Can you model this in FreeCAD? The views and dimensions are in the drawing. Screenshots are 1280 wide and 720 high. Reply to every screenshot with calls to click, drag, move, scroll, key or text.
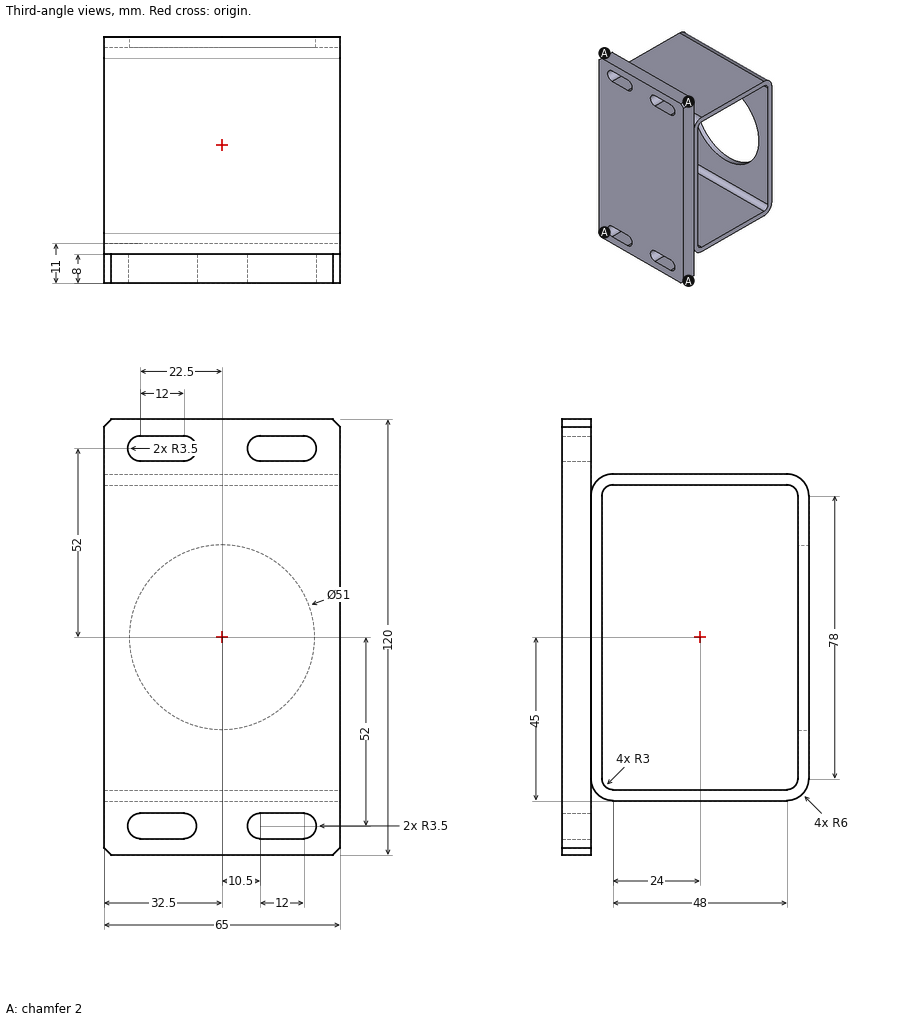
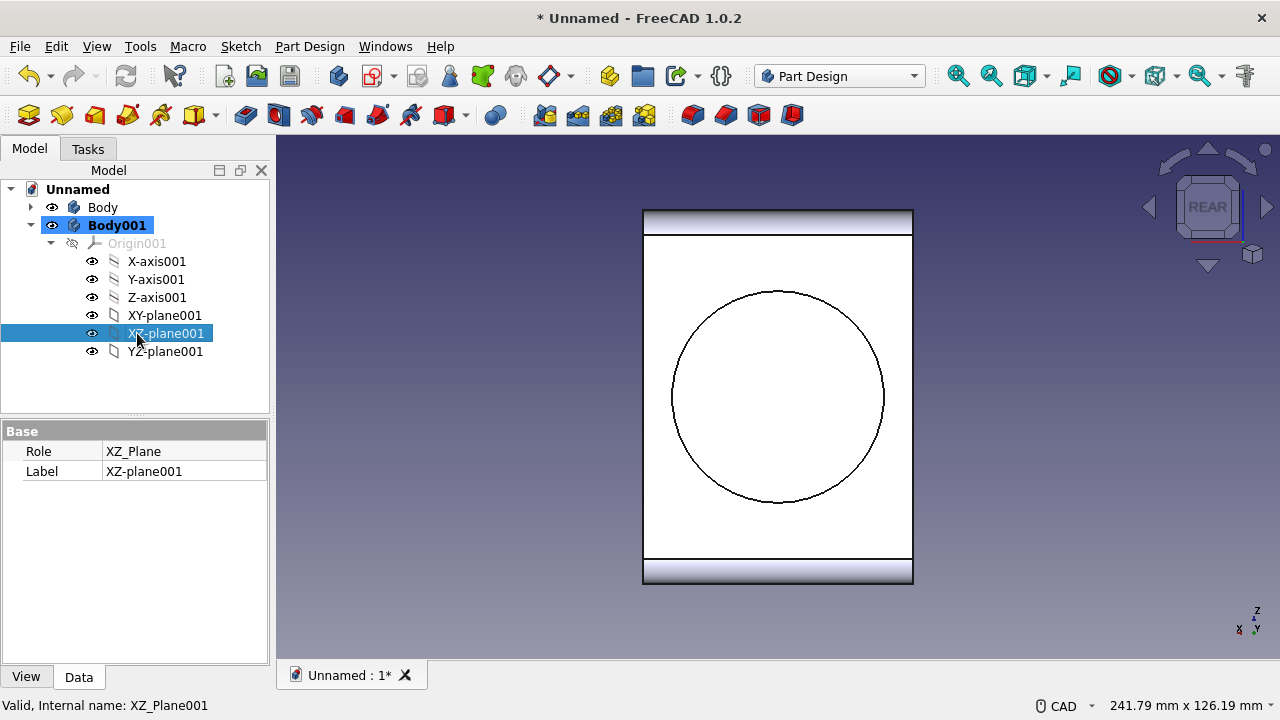
click(548, 76)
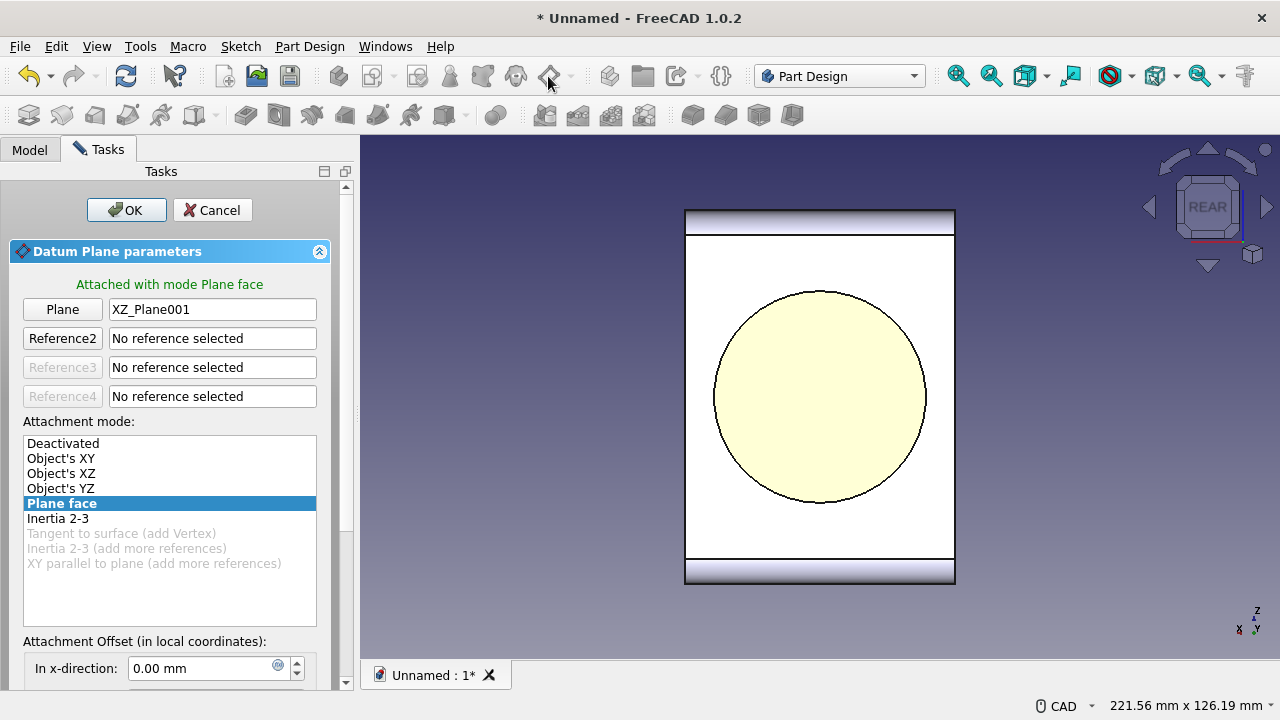
scroll(346, 436, down, 2)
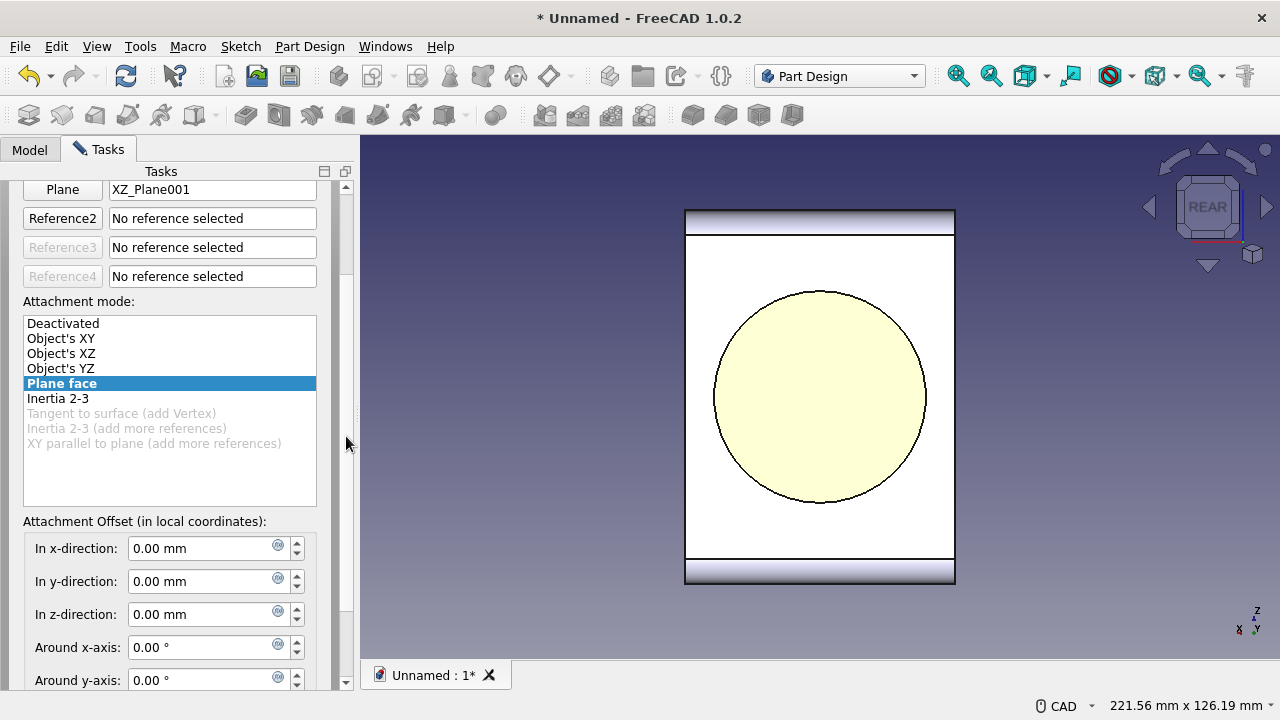
triple_click(210, 614)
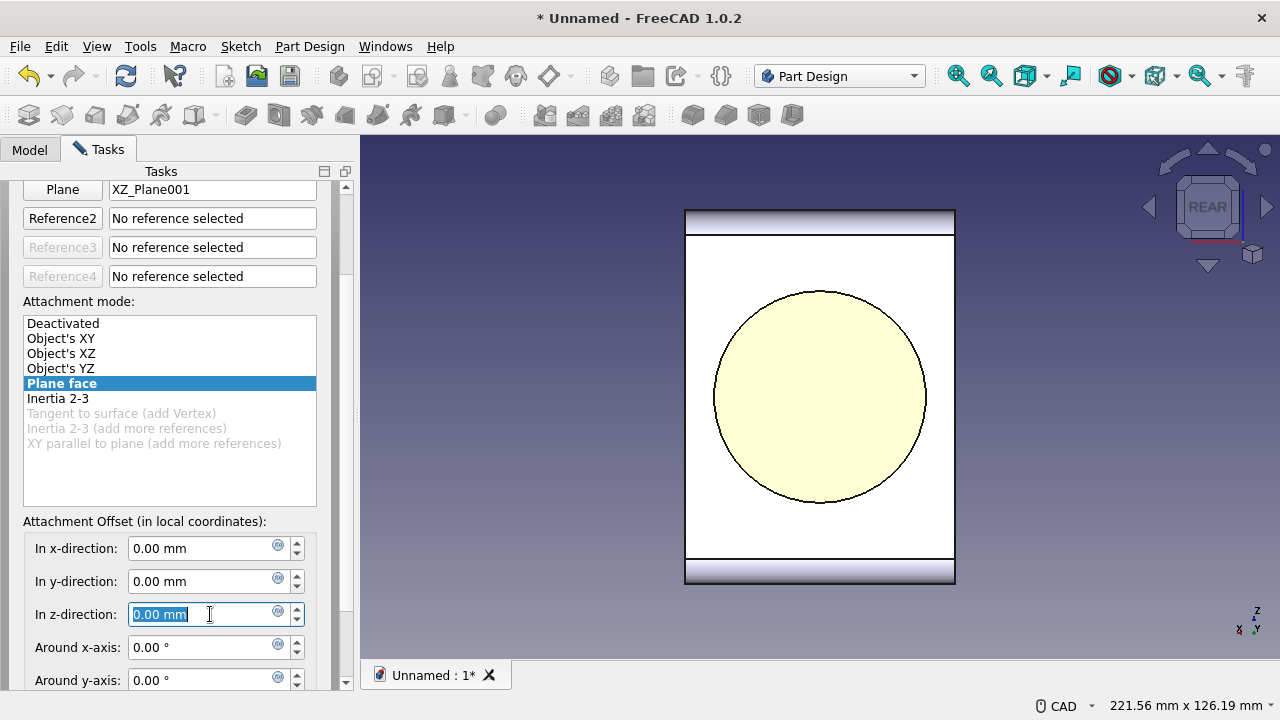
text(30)
key(Tab)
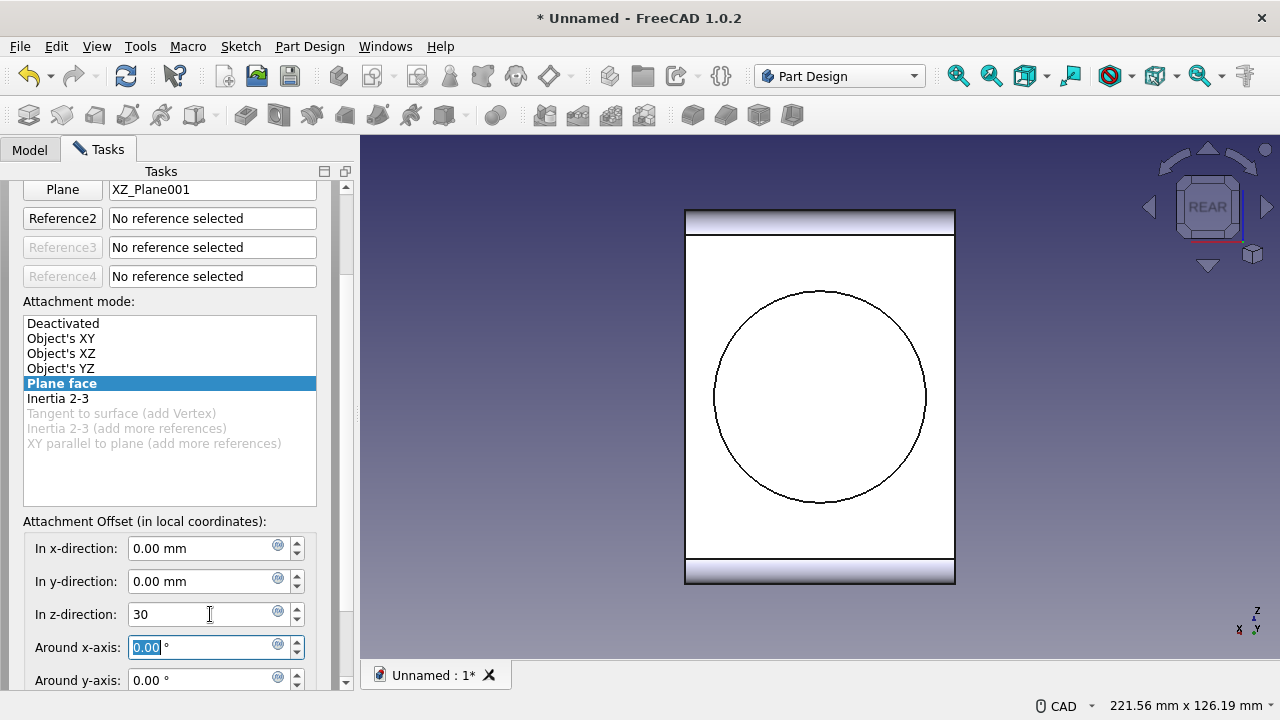
scroll(346, 436, up, 3)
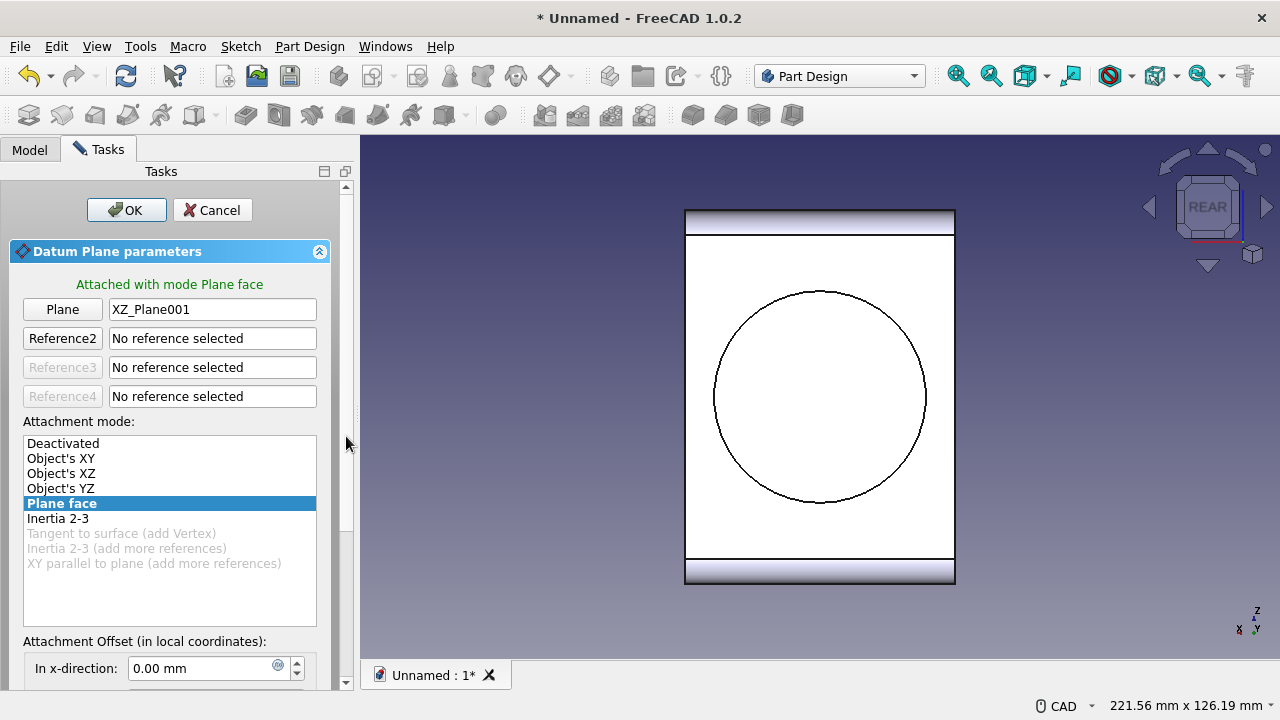
click(127, 210)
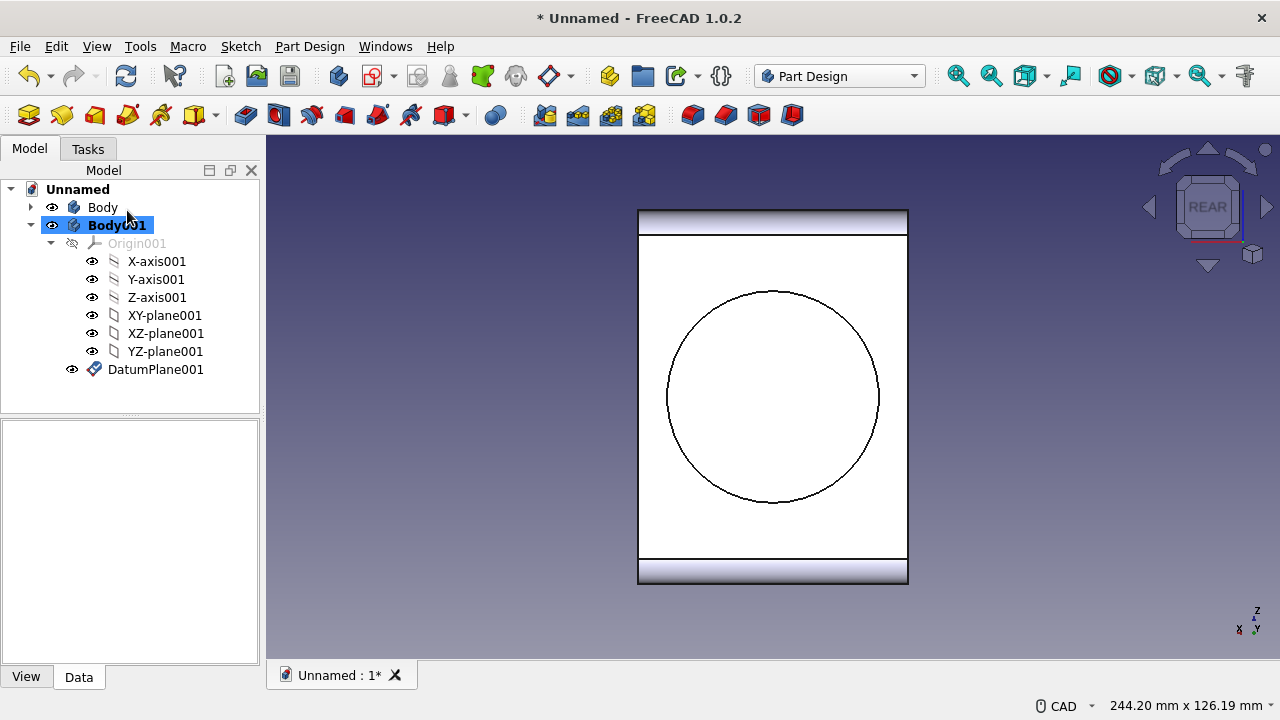
click(117, 369)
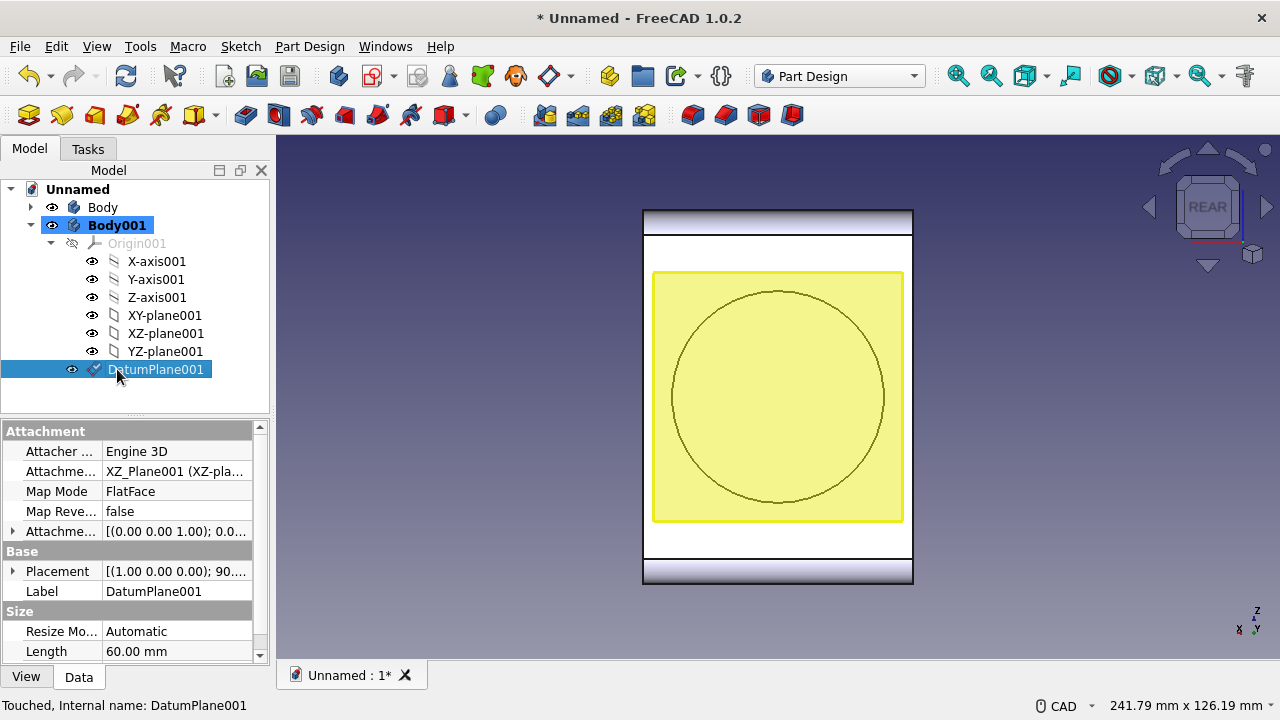
click(372, 76)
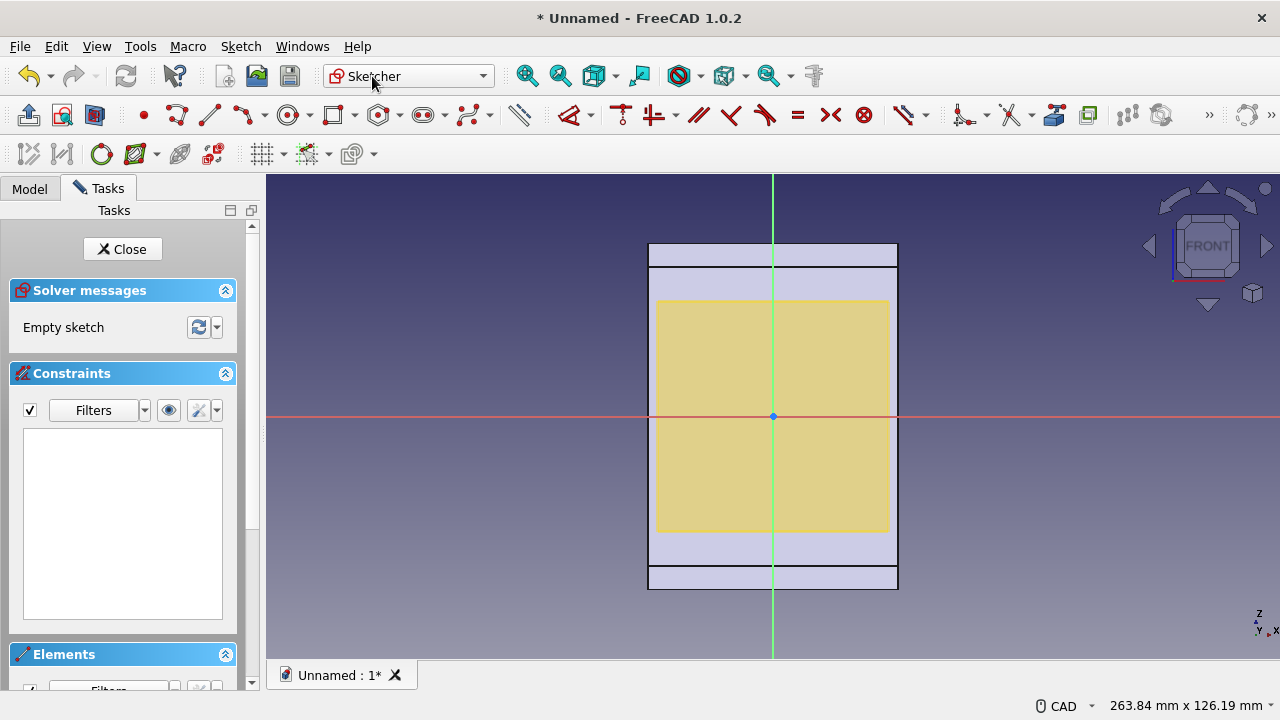
scroll(565, 416, down, 2)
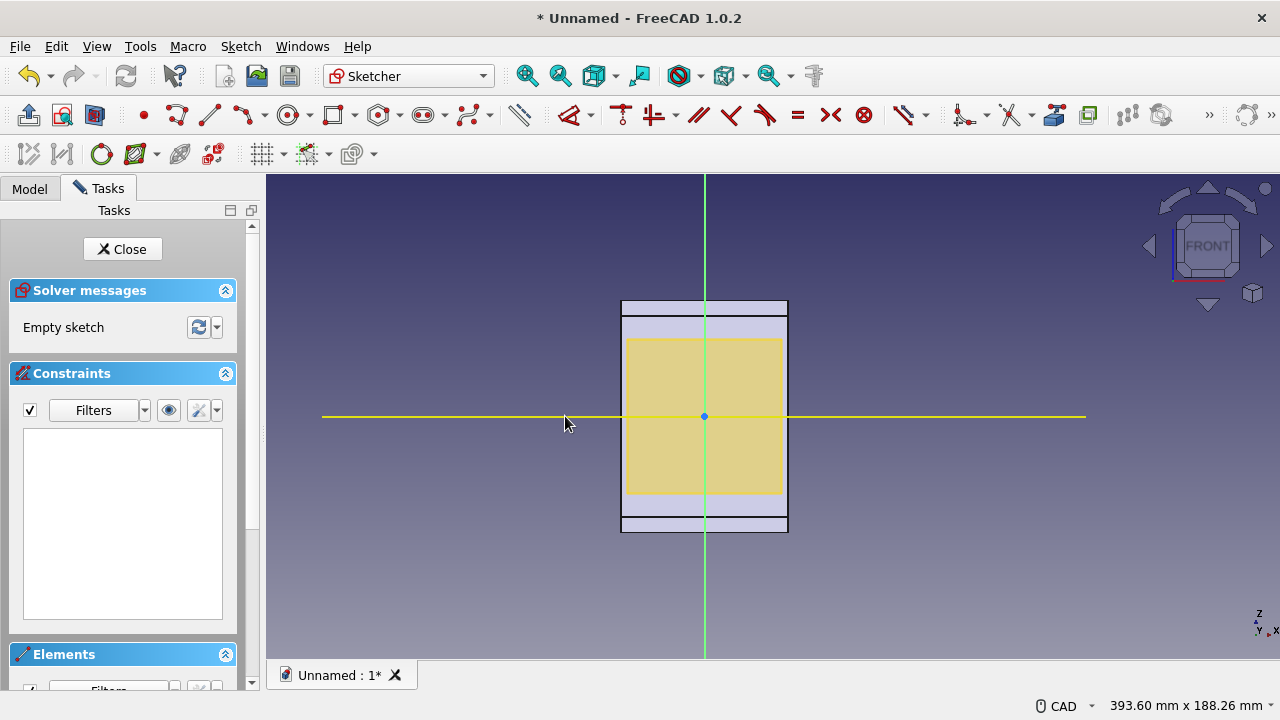
click(354, 116)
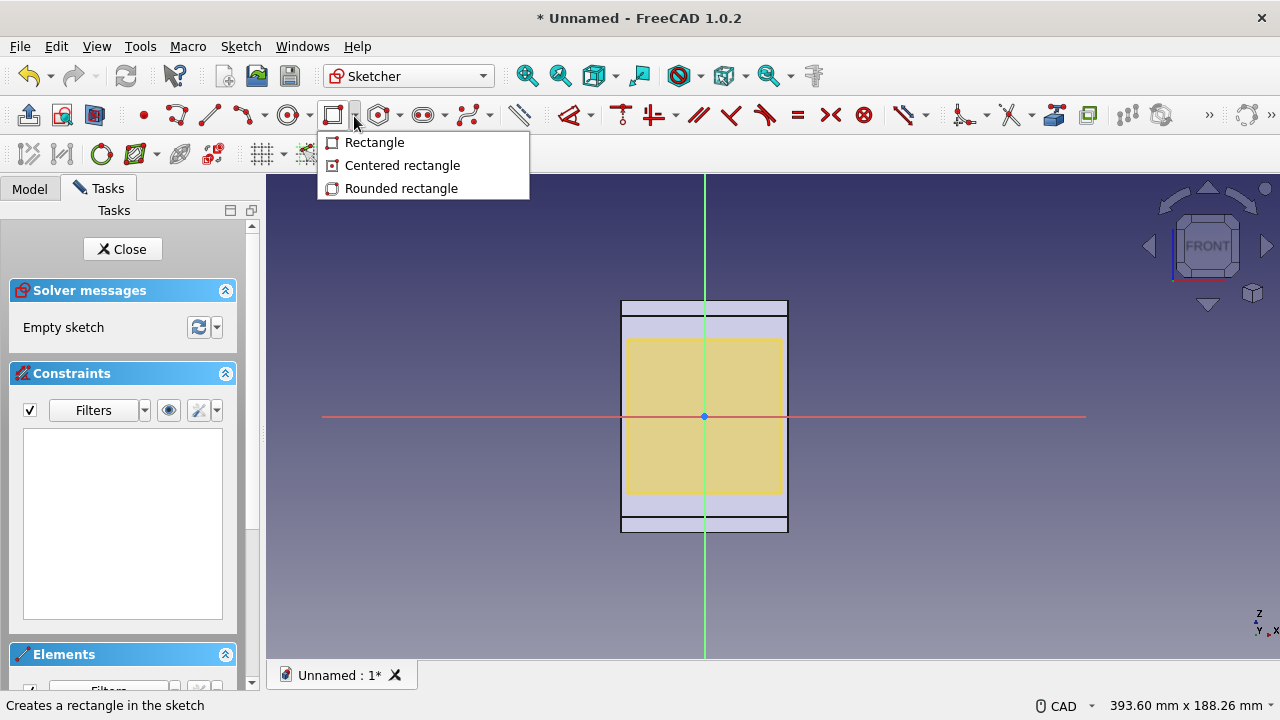
click(424, 166)